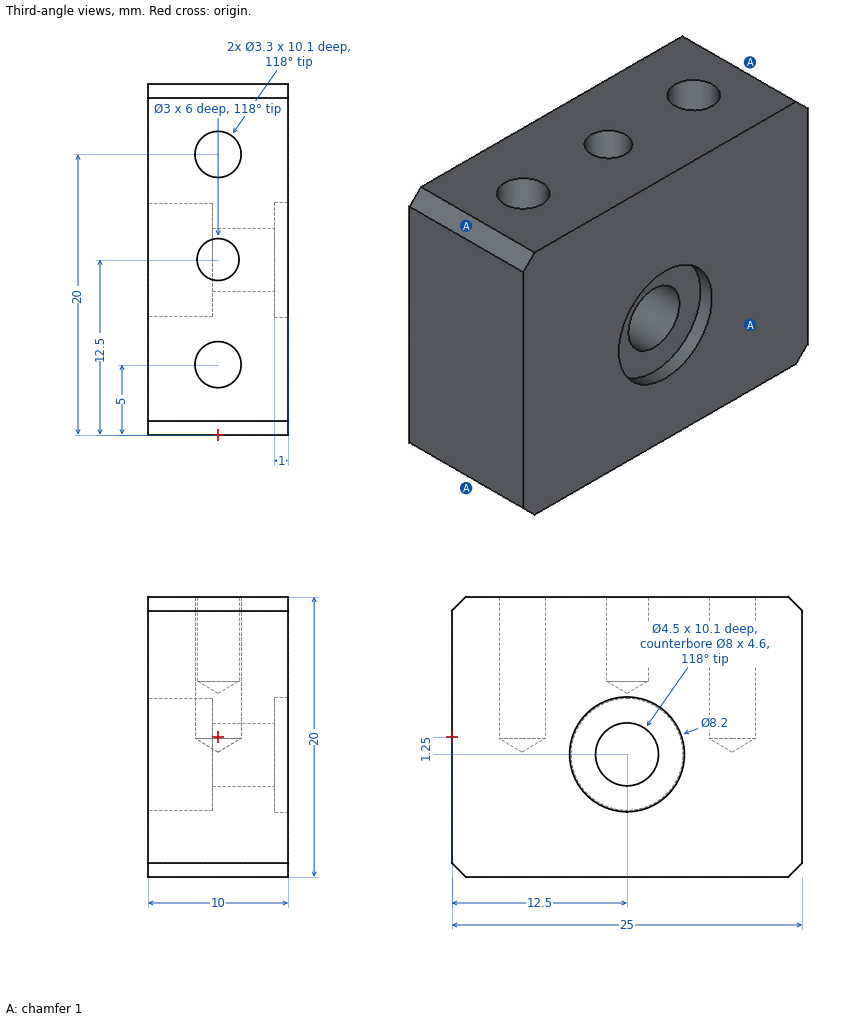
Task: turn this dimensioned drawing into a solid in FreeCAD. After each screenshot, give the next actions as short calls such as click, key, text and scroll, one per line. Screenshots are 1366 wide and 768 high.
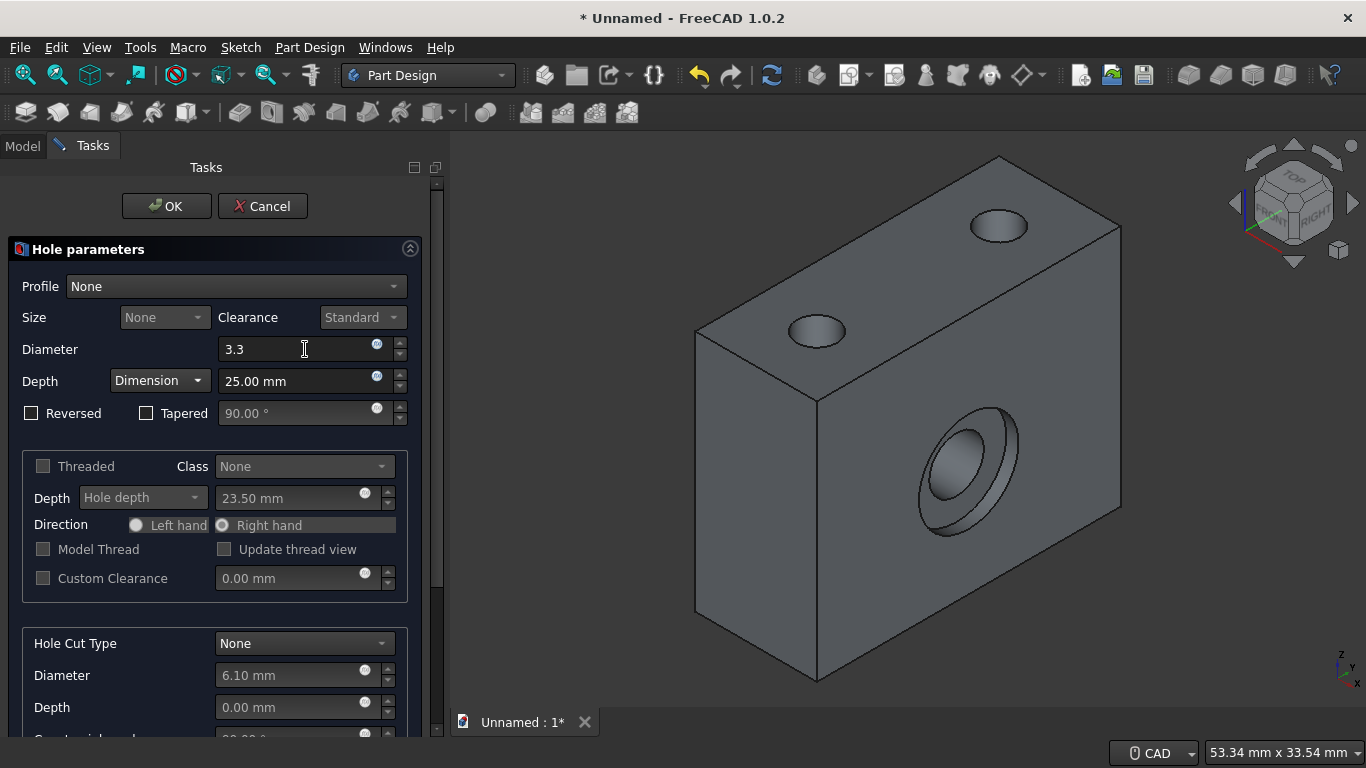
triple_click(305, 381)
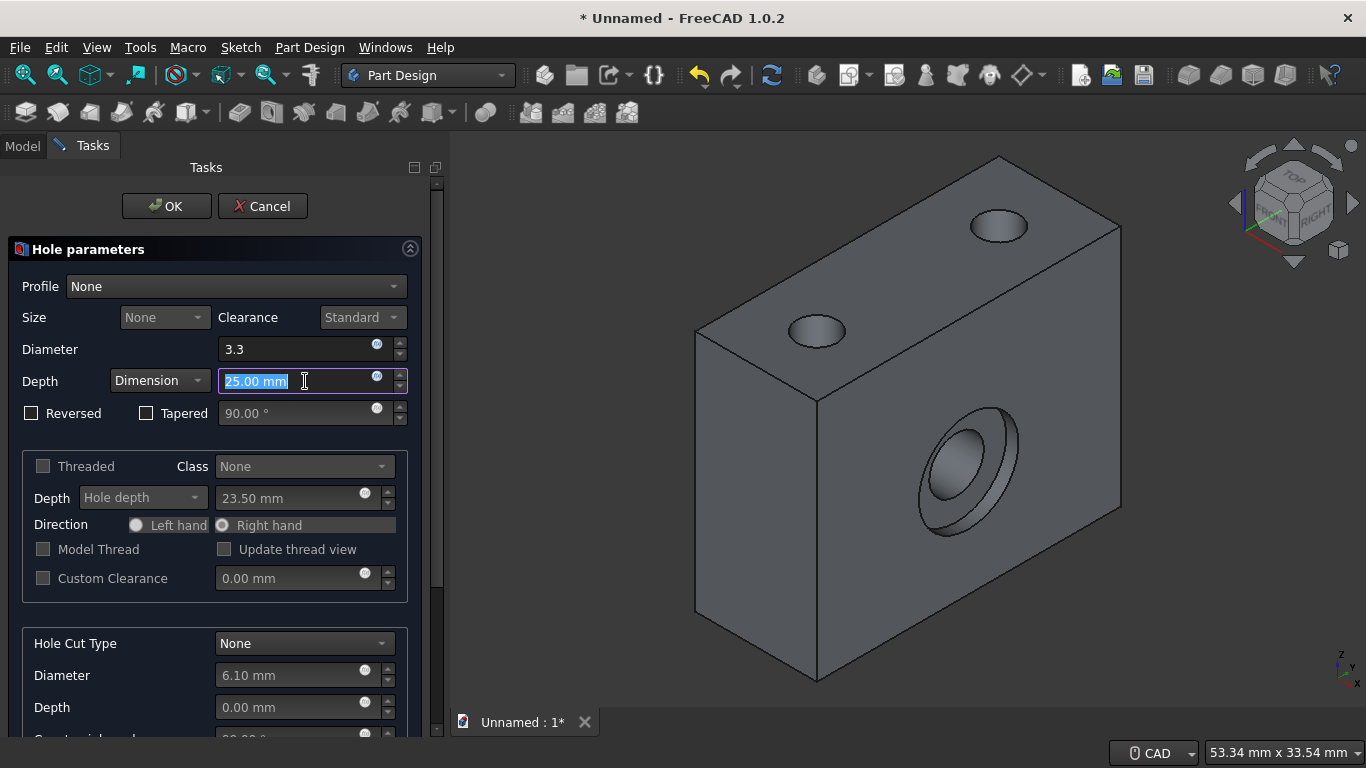
text(10.1)
key(Tab)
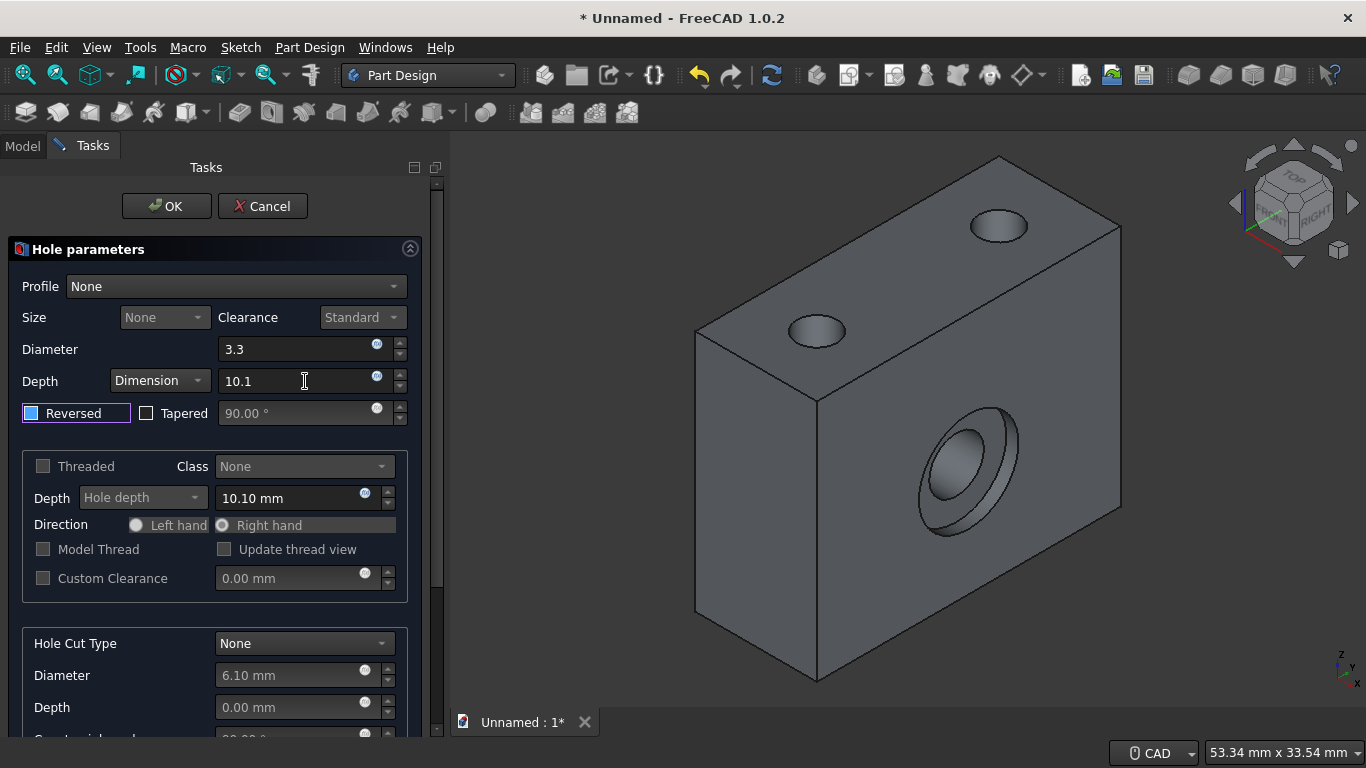
click(167, 206)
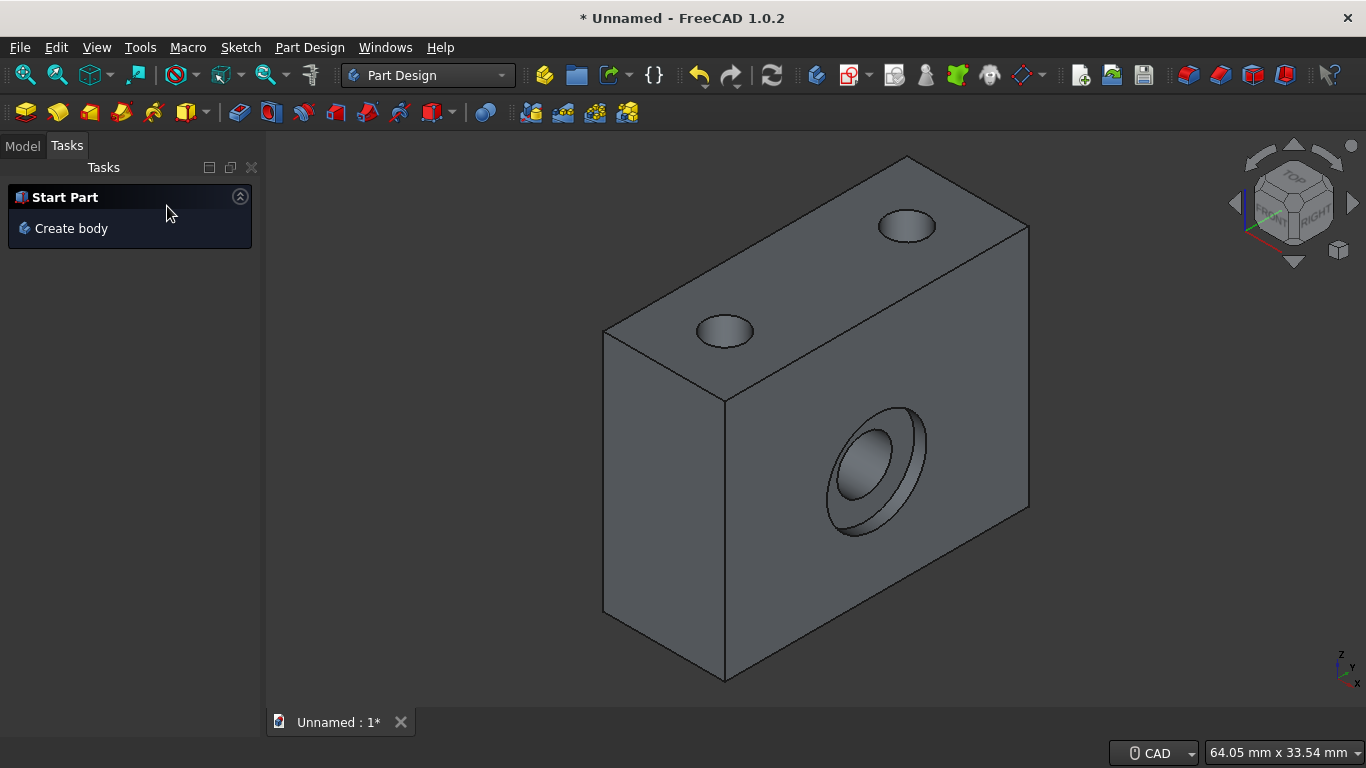
click(816, 278)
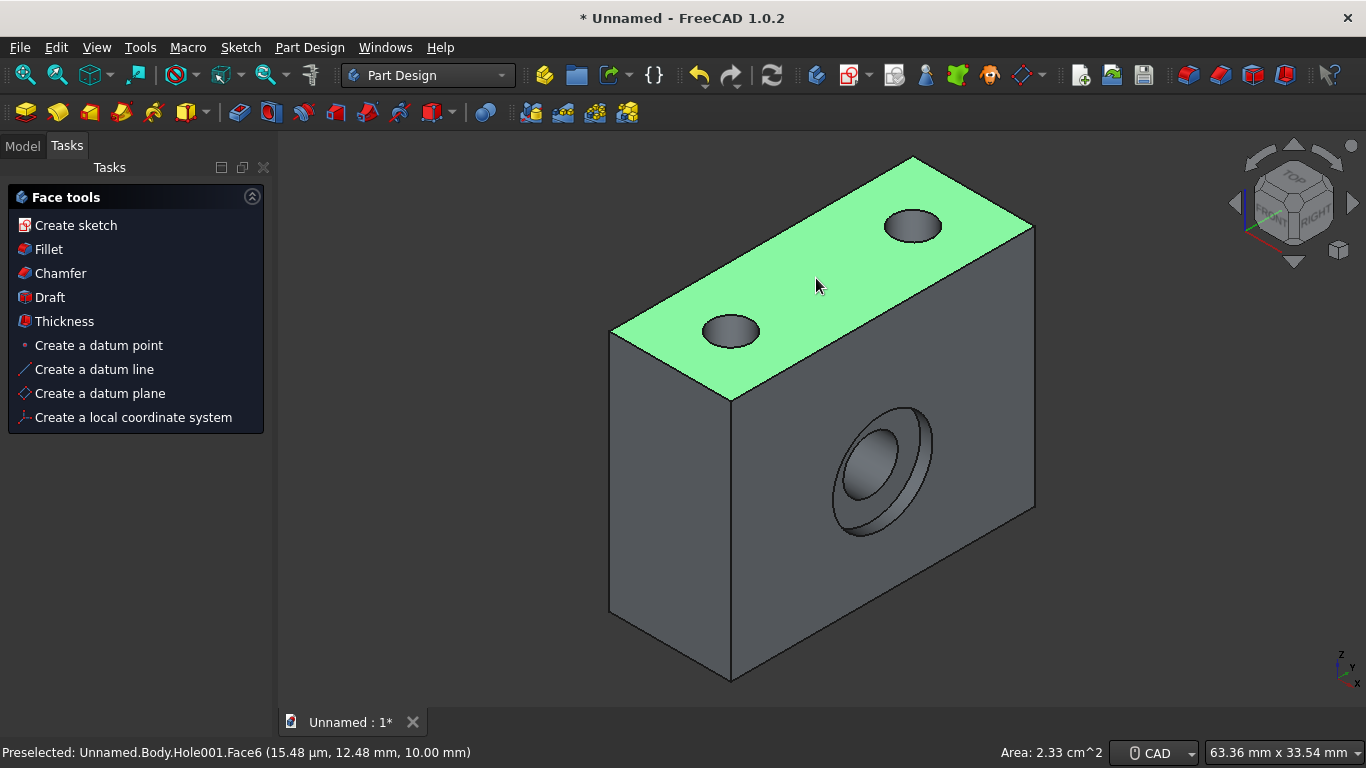
click(850, 76)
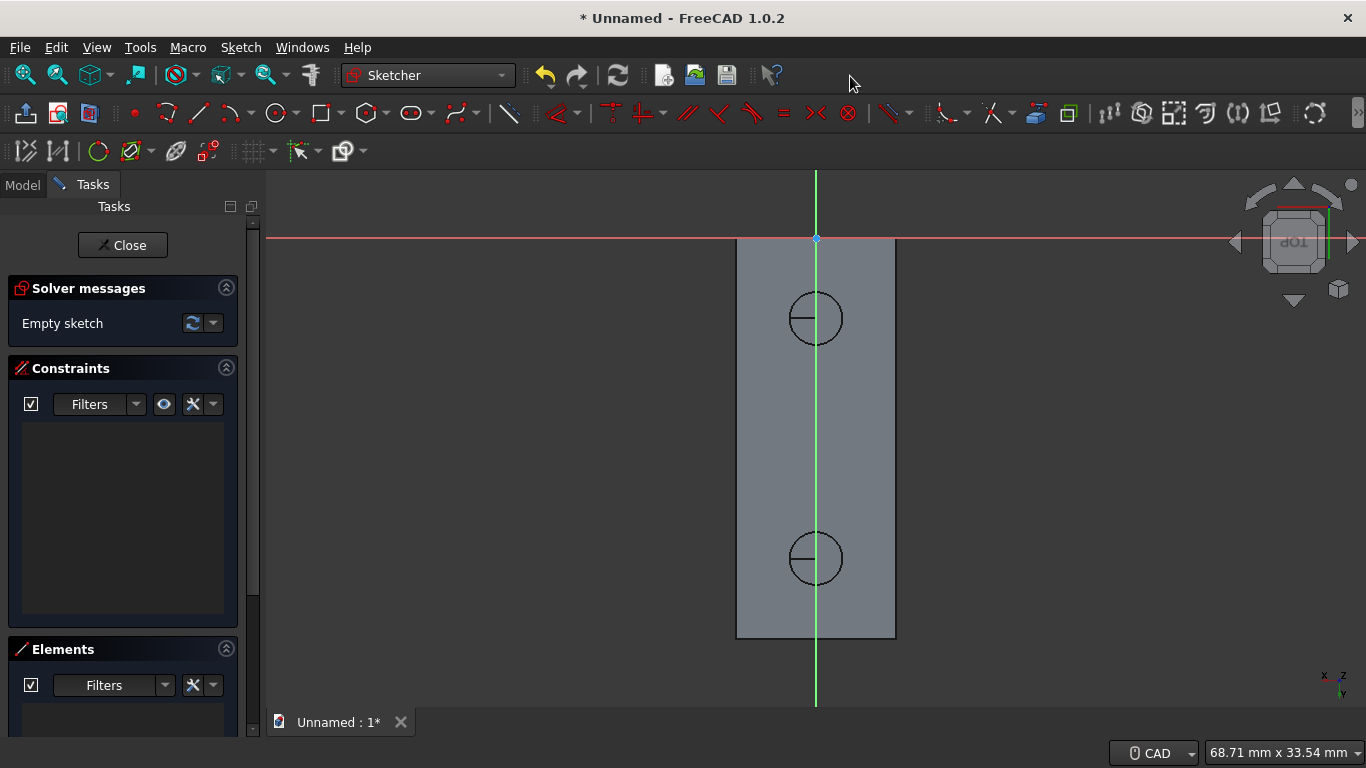
scroll(827, 438, up, 10)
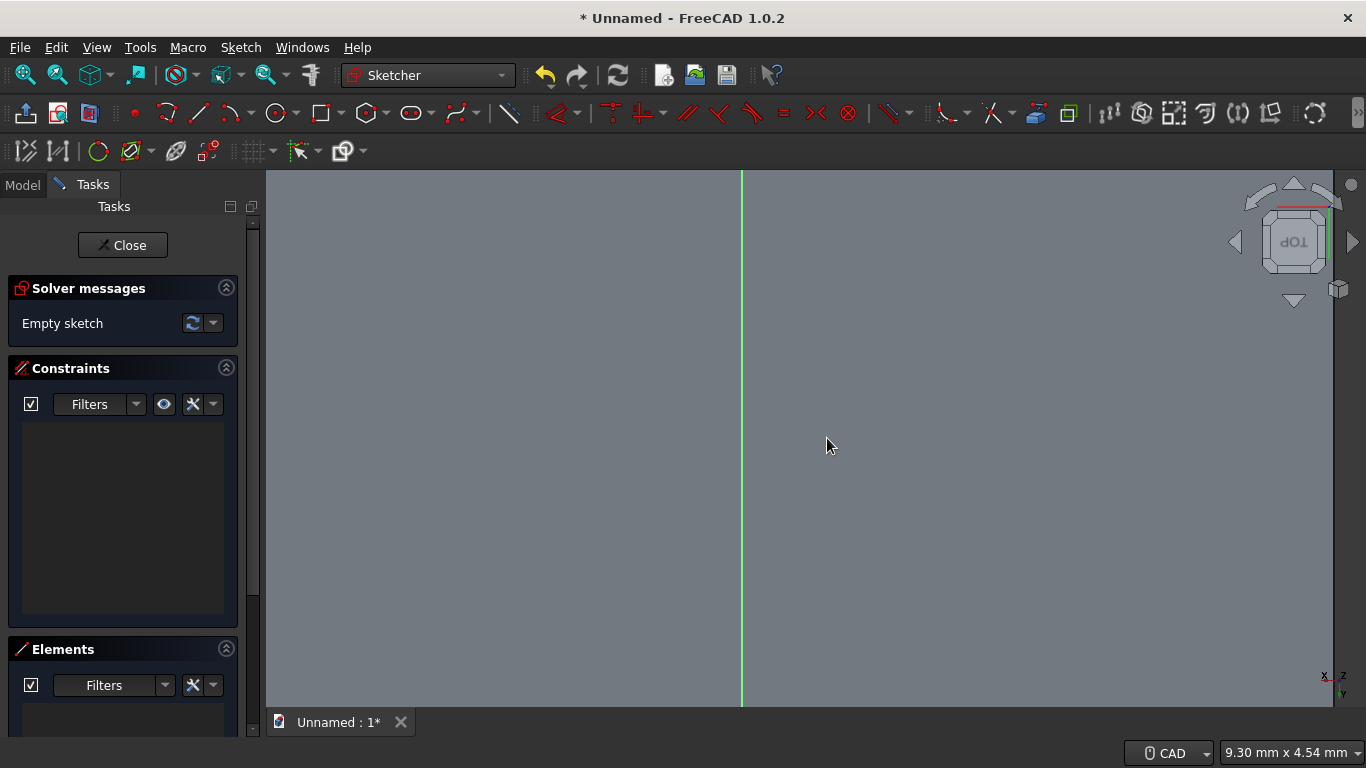
click(276, 114)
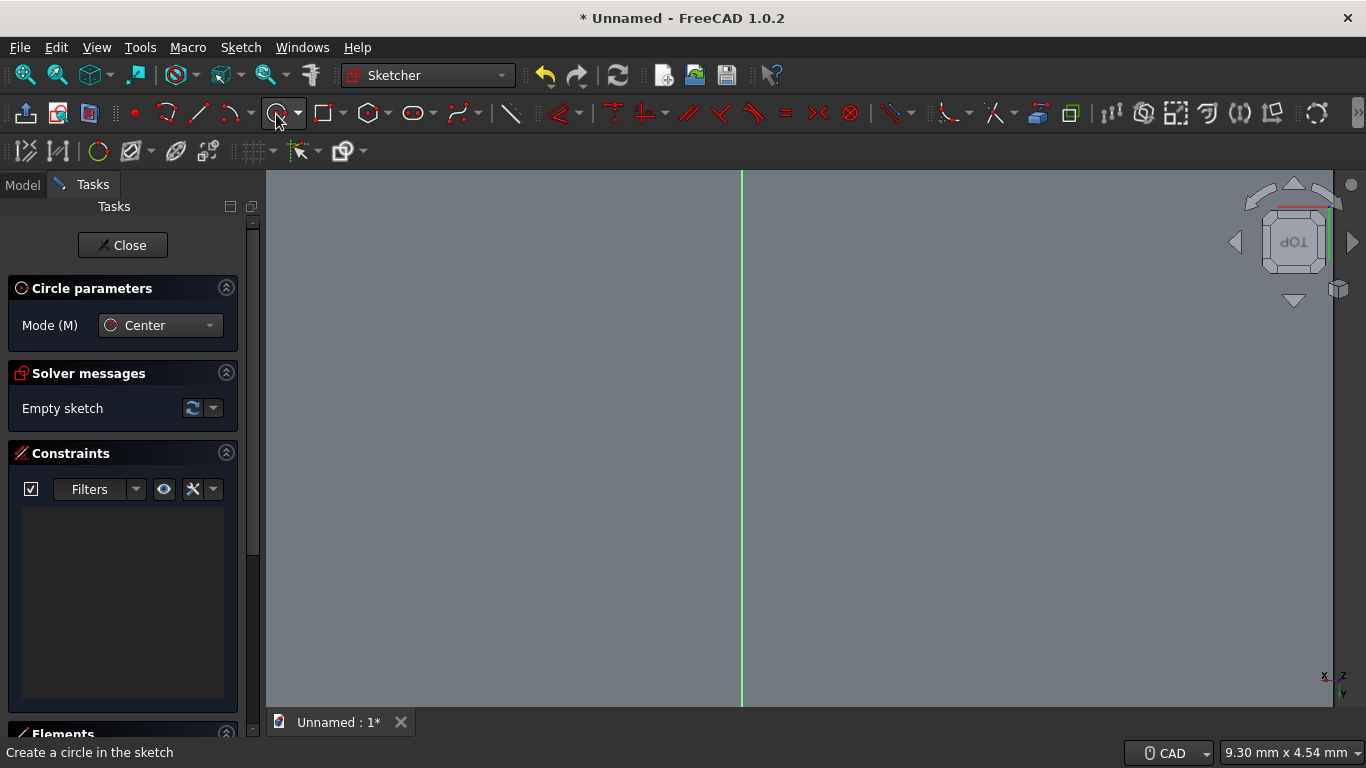
click(742, 438)
click(868, 313)
key(Escape)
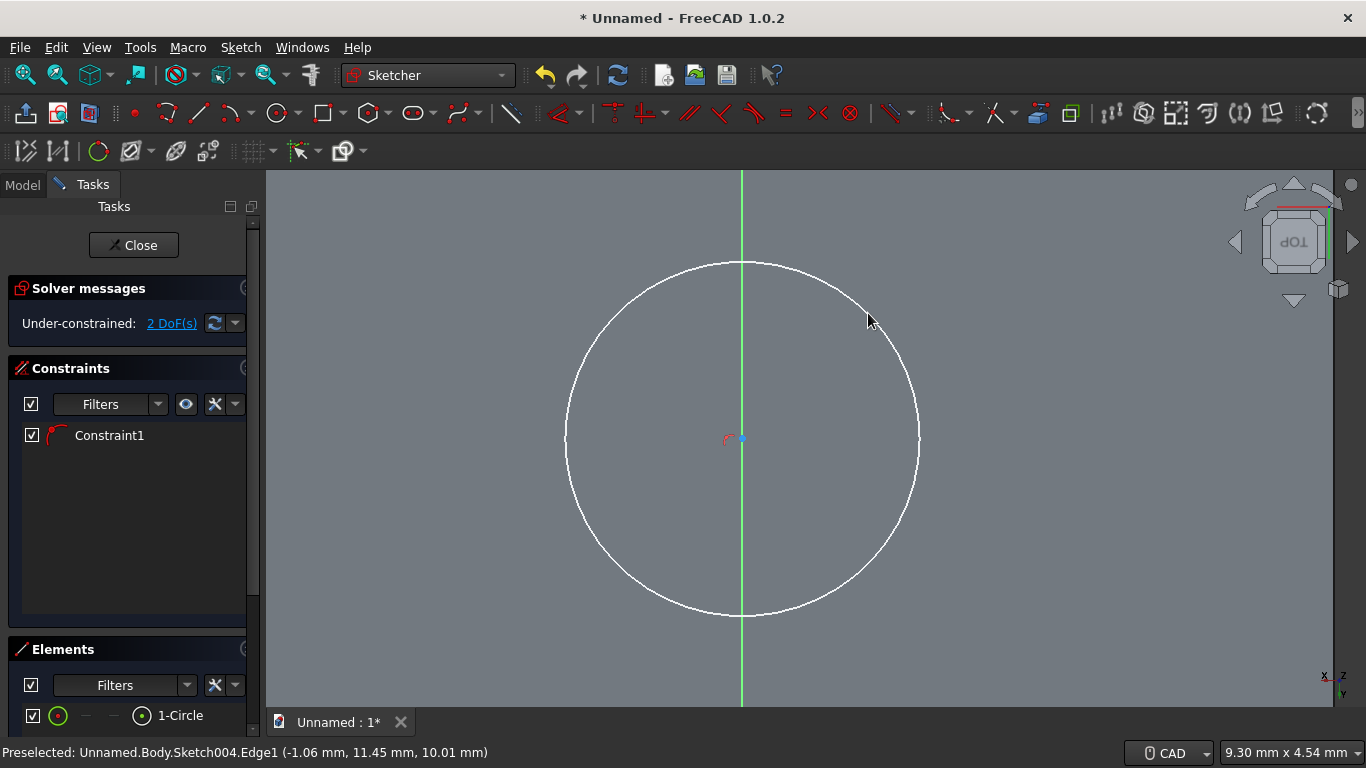
click(558, 114)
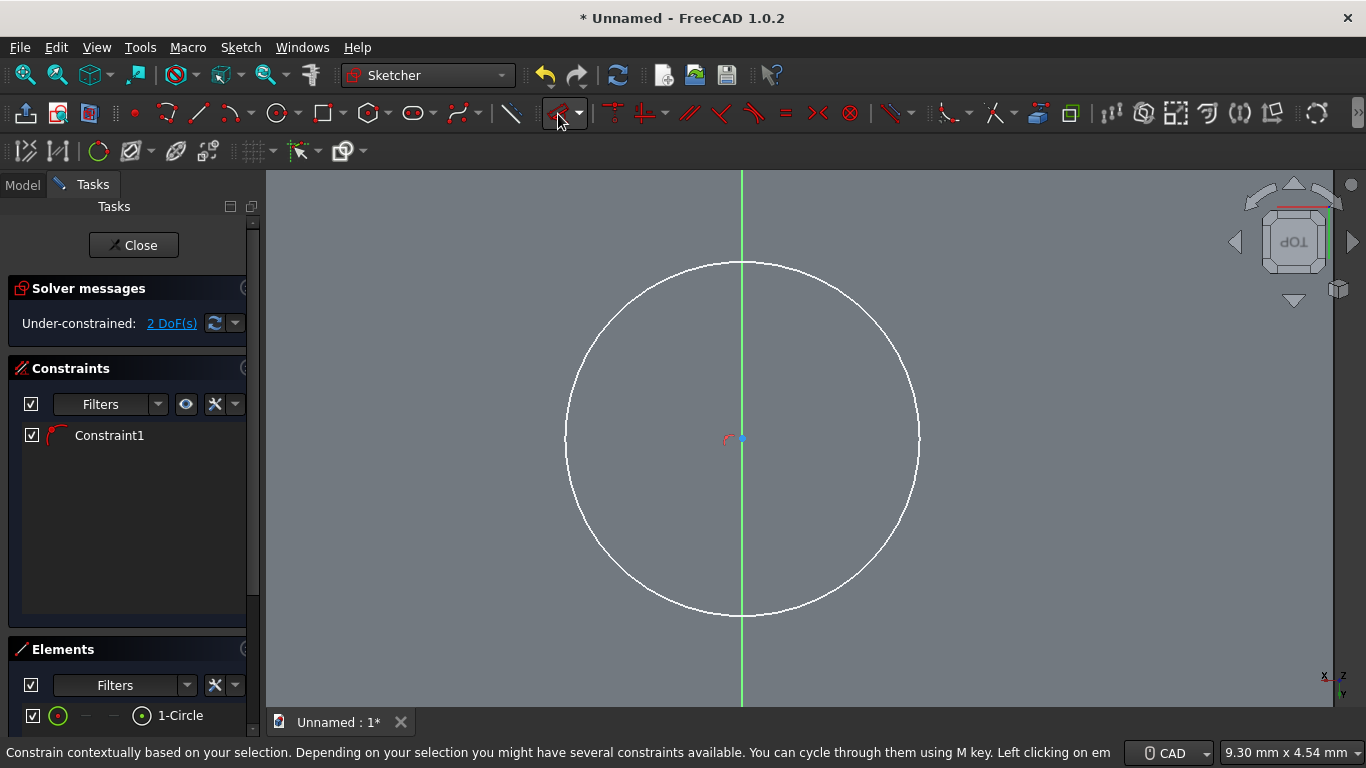
click(867, 313)
click(889, 290)